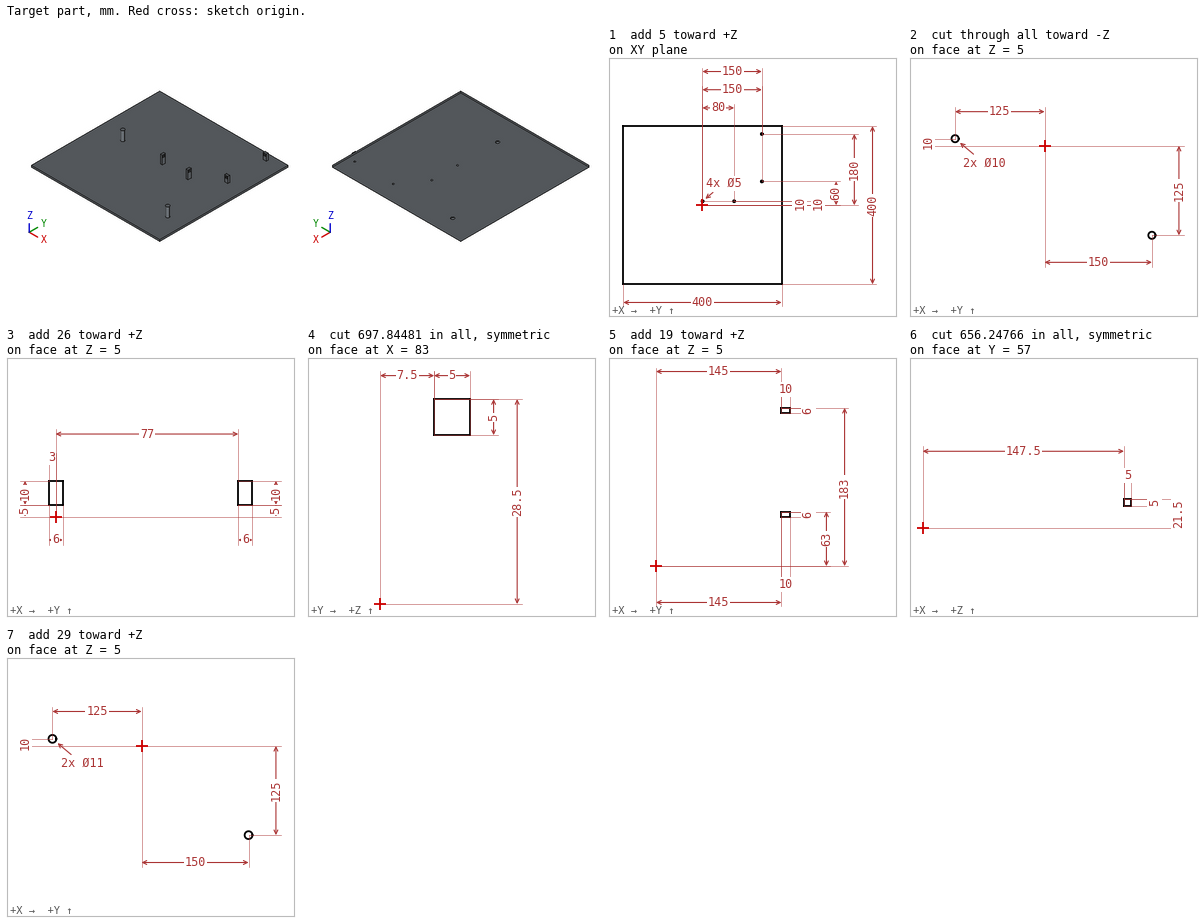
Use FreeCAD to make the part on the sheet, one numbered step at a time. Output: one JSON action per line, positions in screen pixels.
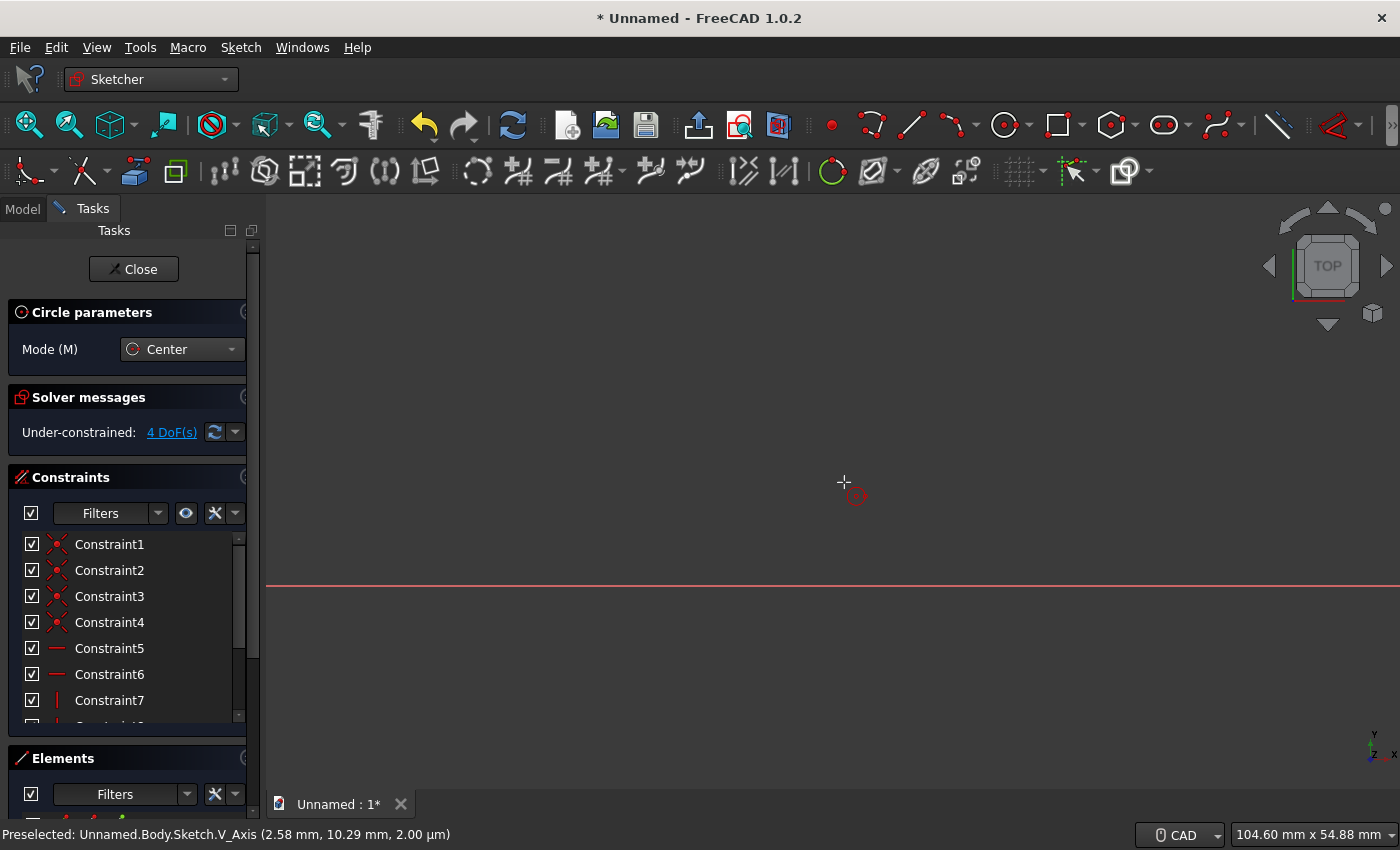
{"action": "scroll", "coordinate": [844, 482], "scroll_direction": "down", "scroll_amount": 12}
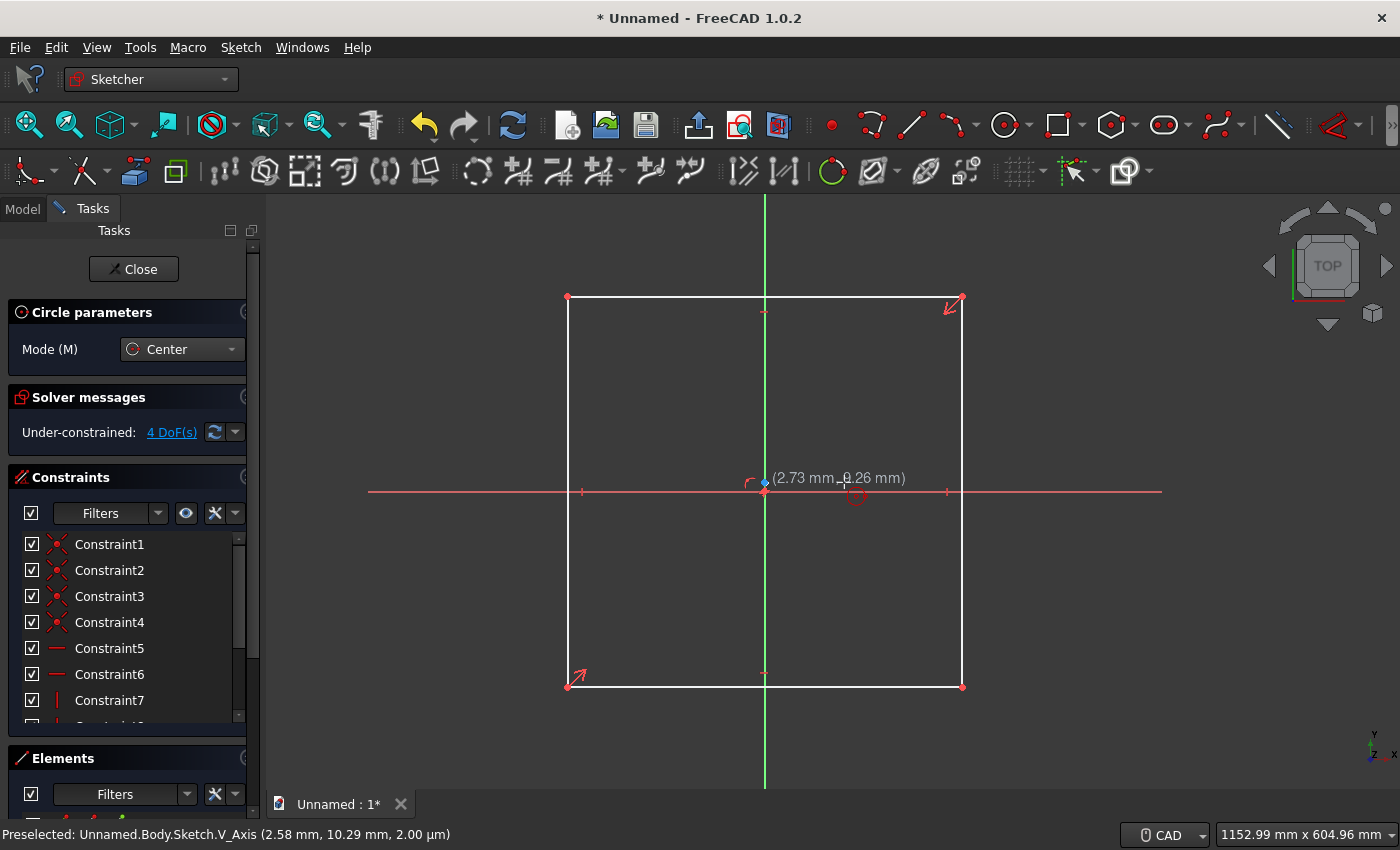
{"action": "scroll", "coordinate": [844, 482], "scroll_direction": "up", "scroll_amount": 3}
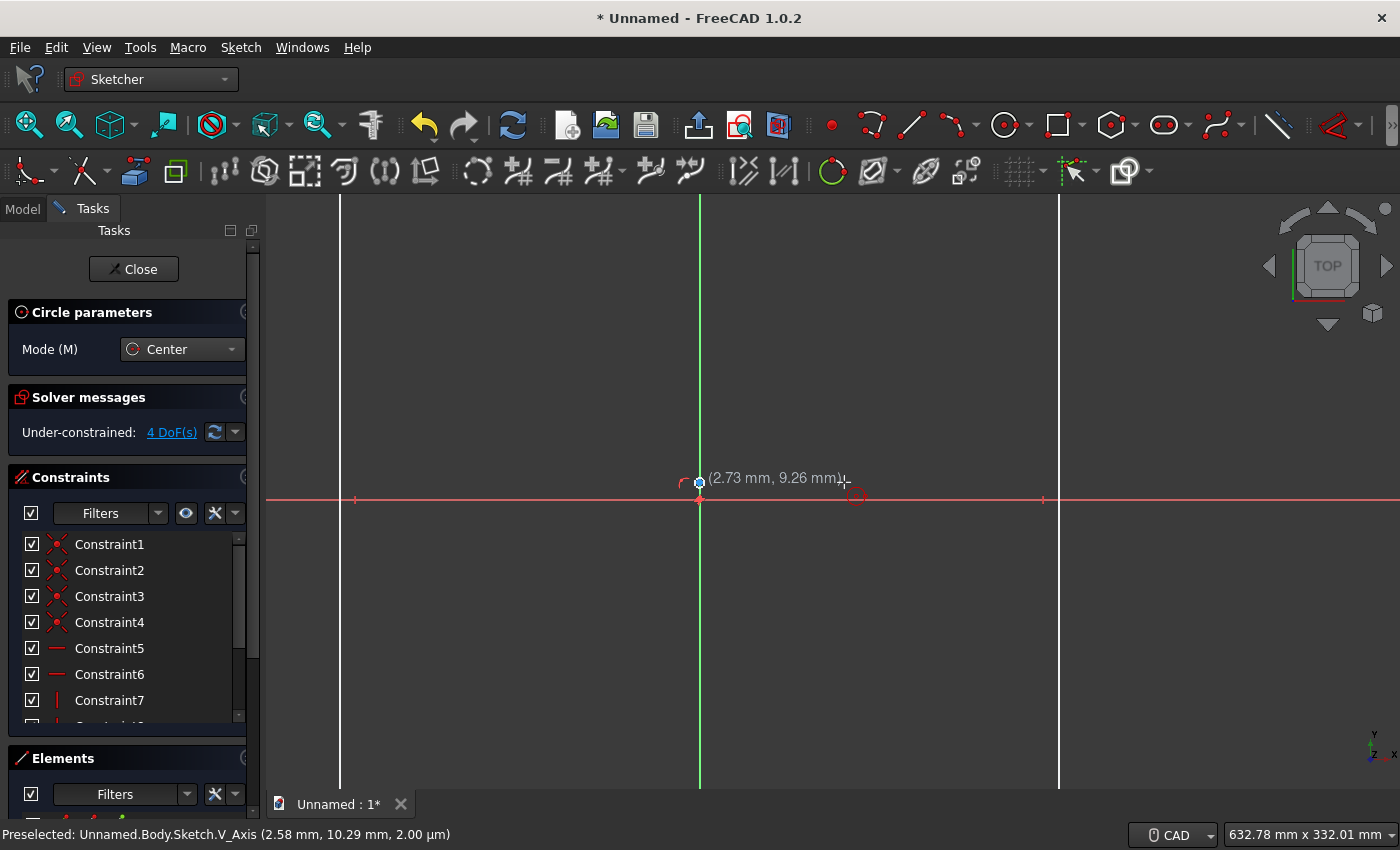
{"action": "left_click", "coordinate": [843, 482]}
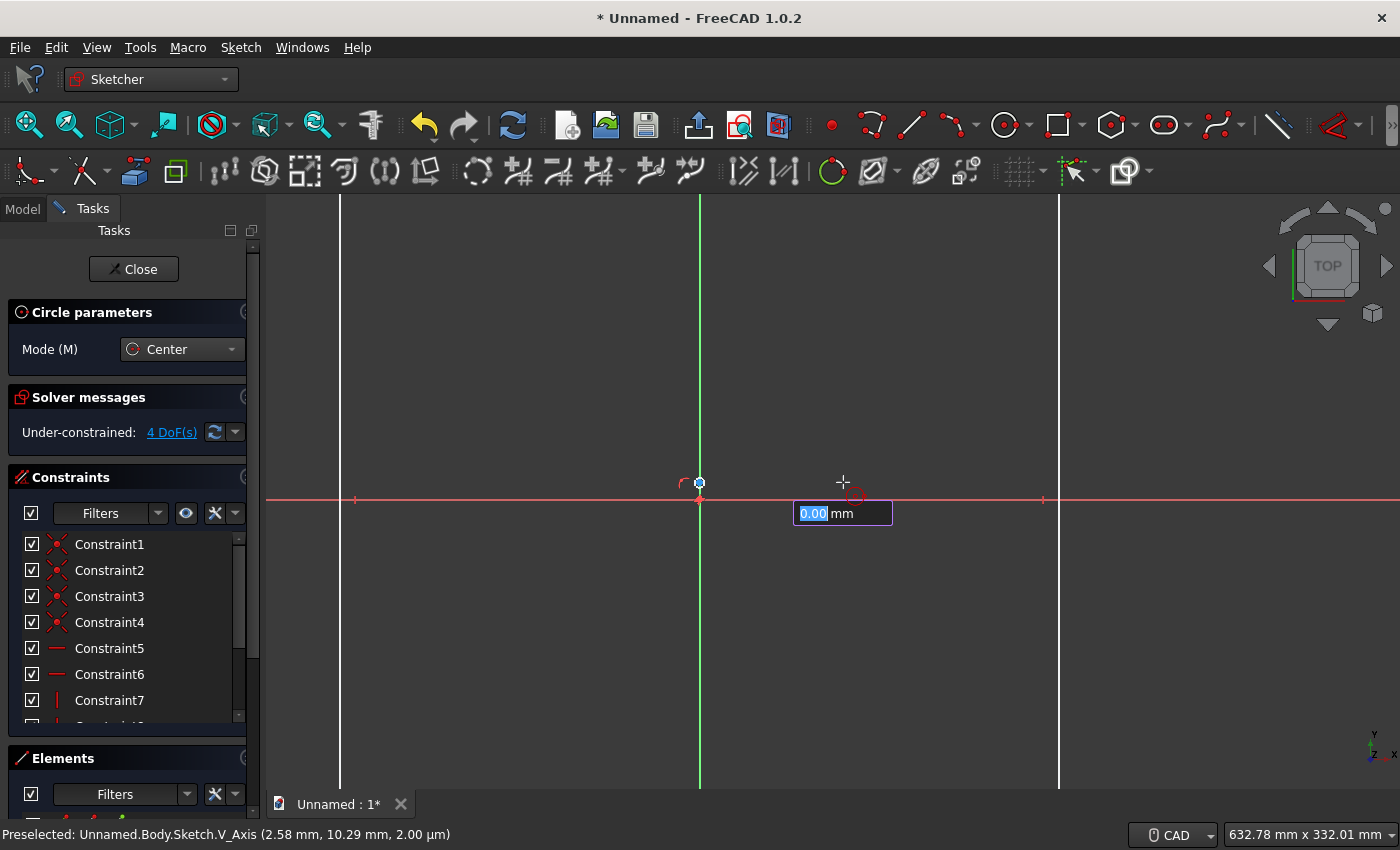
{"action": "scroll", "coordinate": [846, 478], "scroll_direction": "up", "scroll_amount": 7}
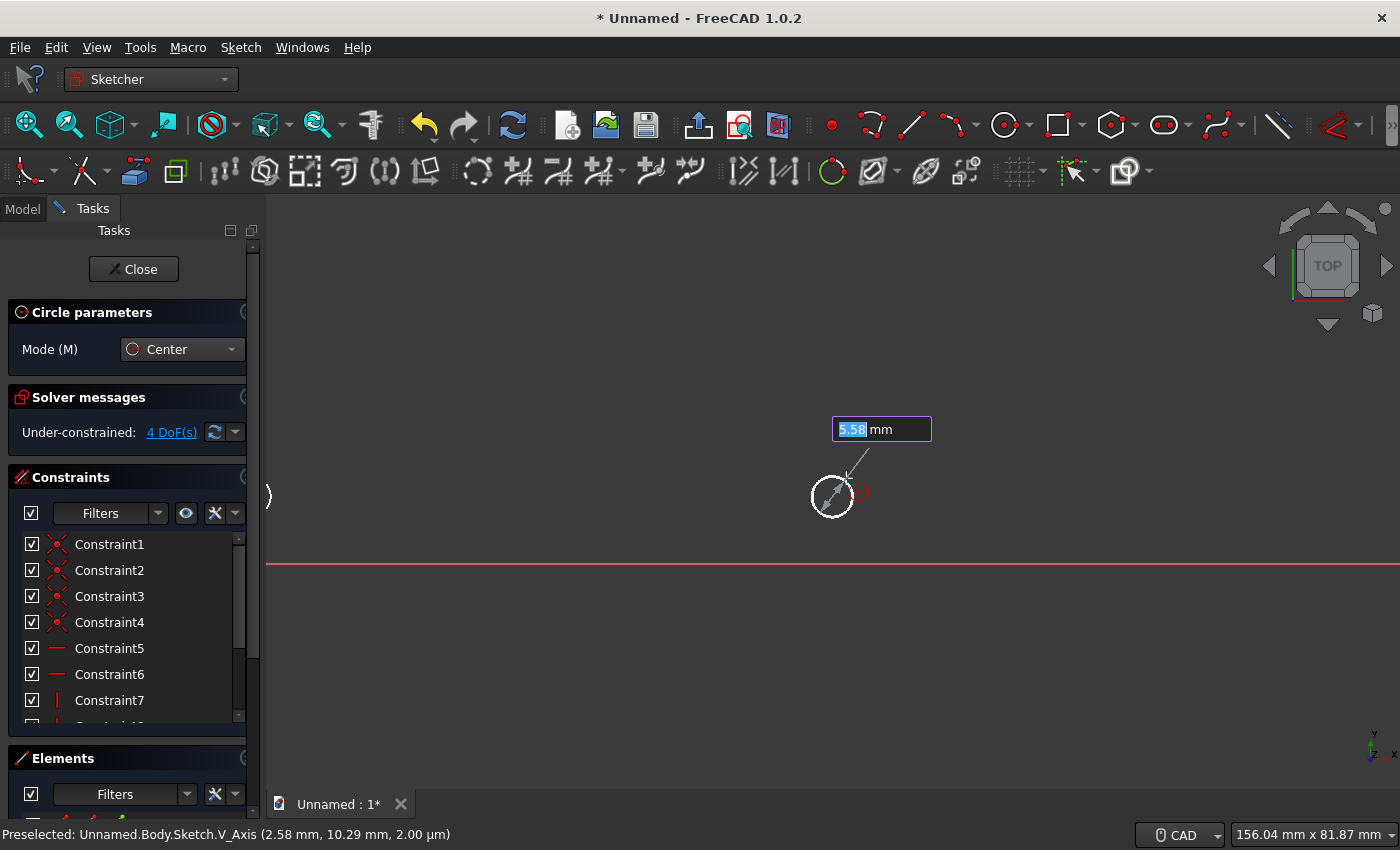
{"action": "left_click", "coordinate": [845, 478]}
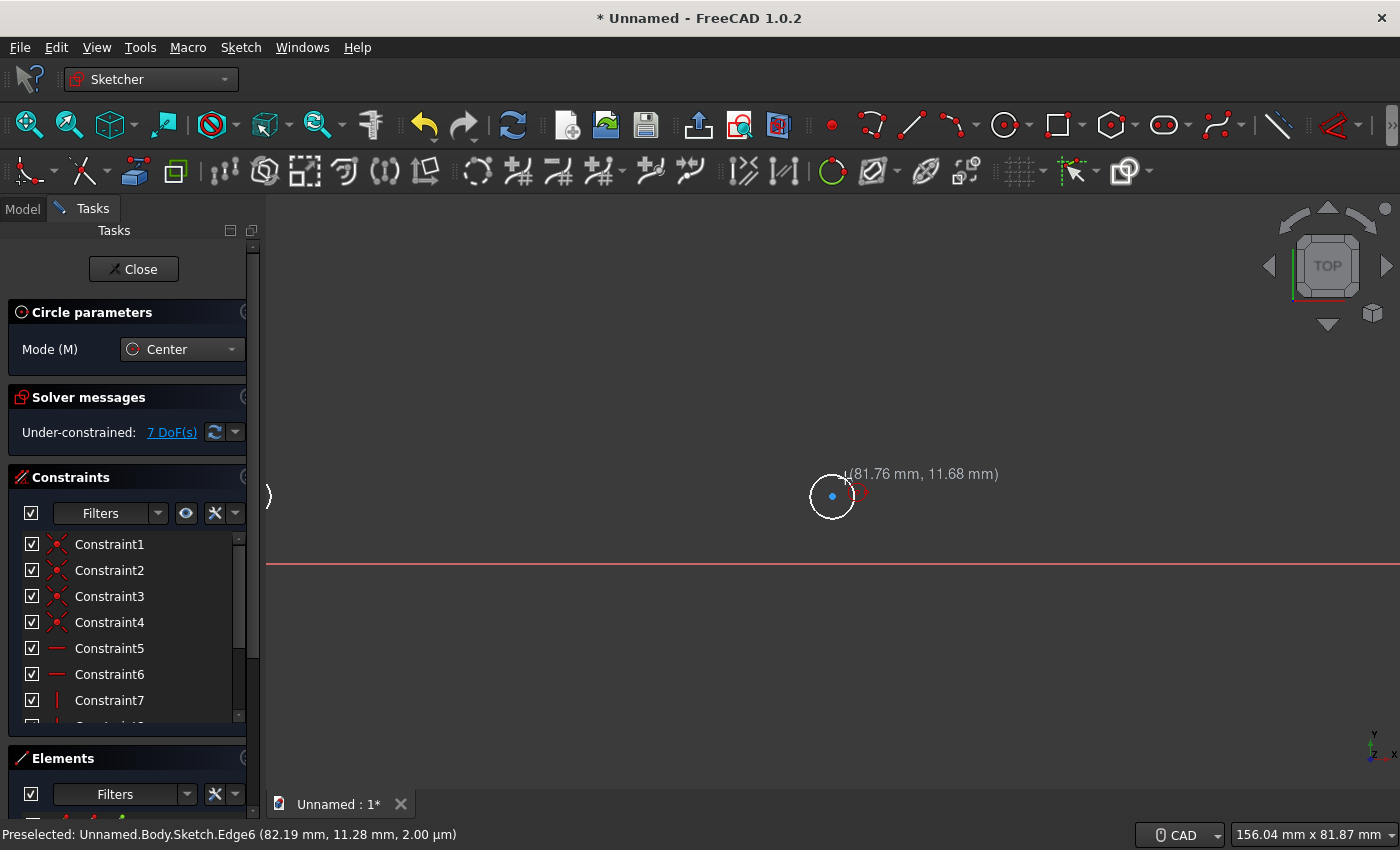
{"action": "scroll", "coordinate": [845, 480], "scroll_direction": "down", "scroll_amount": 10}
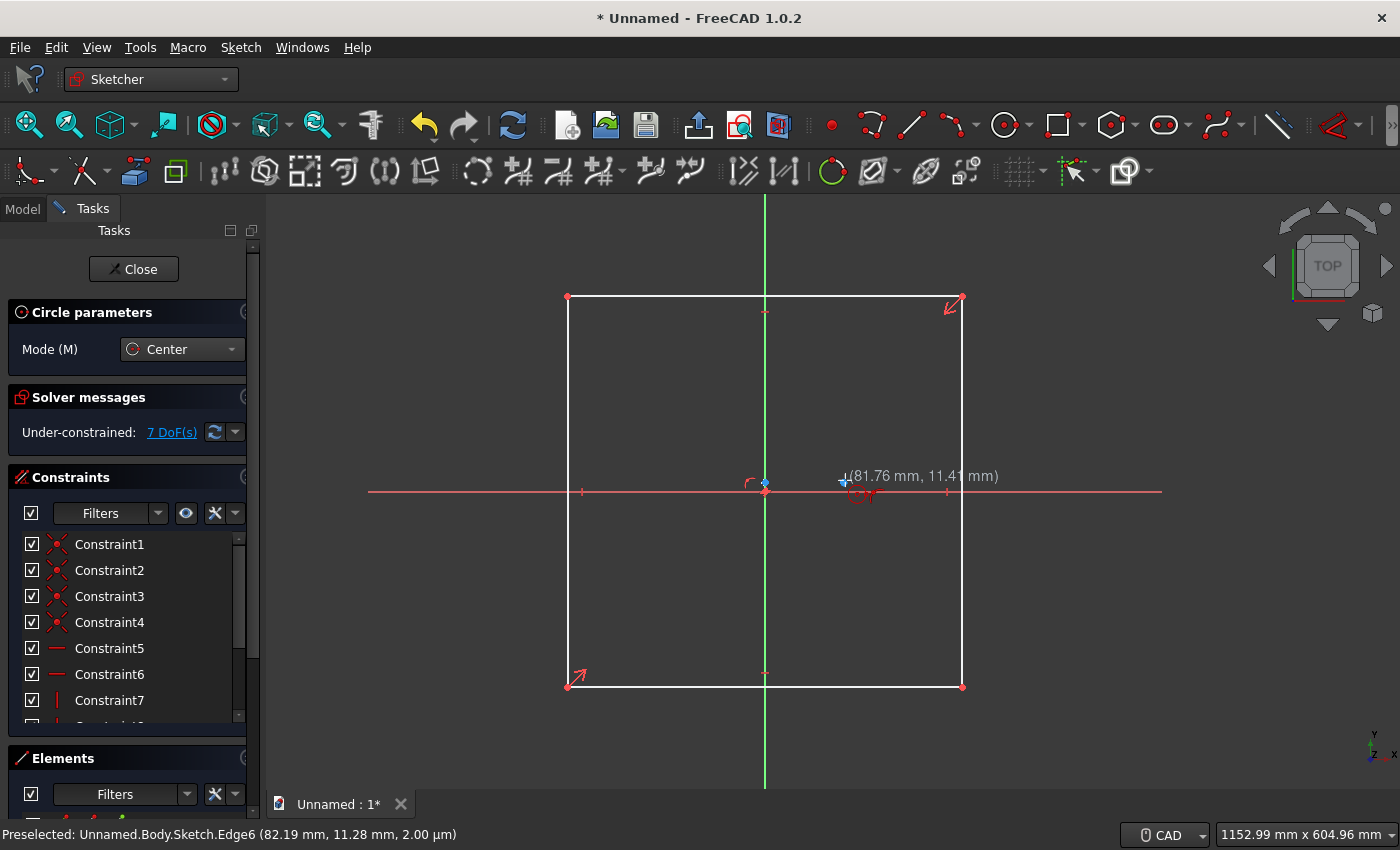
{"action": "scroll", "coordinate": [913, 433], "scroll_direction": "up", "scroll_amount": 12}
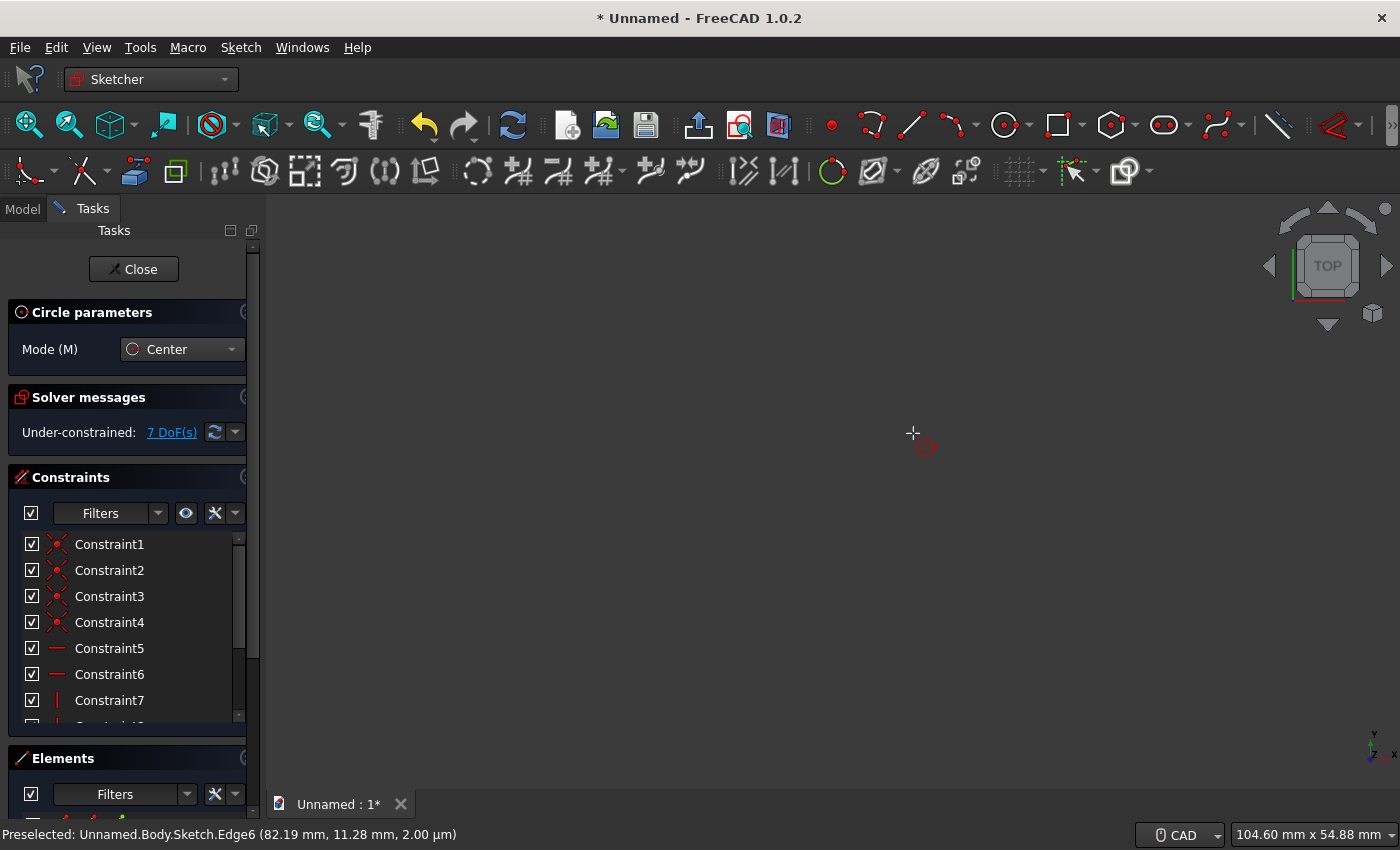
{"action": "scroll", "coordinate": [913, 433], "scroll_direction": "down", "scroll_amount": 12}